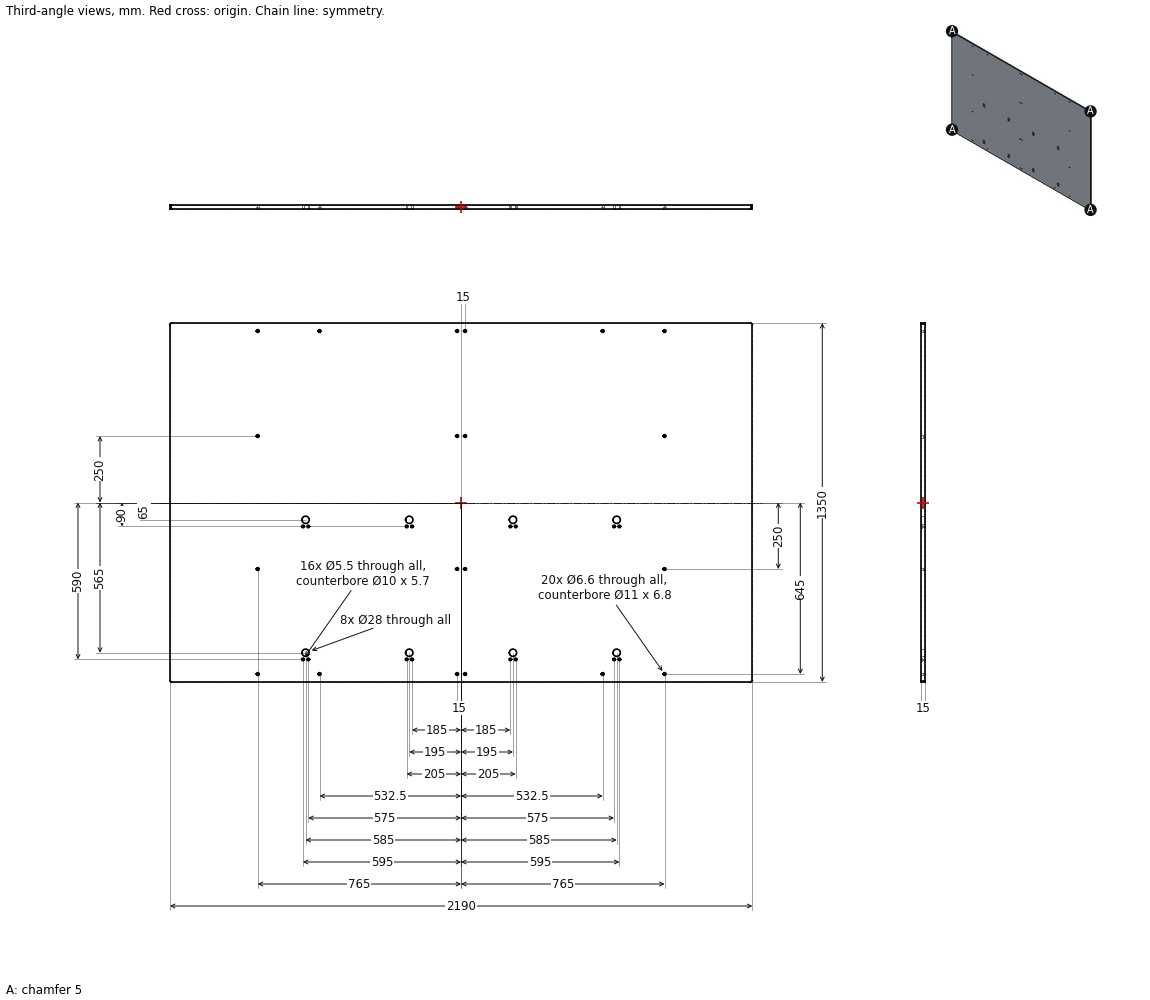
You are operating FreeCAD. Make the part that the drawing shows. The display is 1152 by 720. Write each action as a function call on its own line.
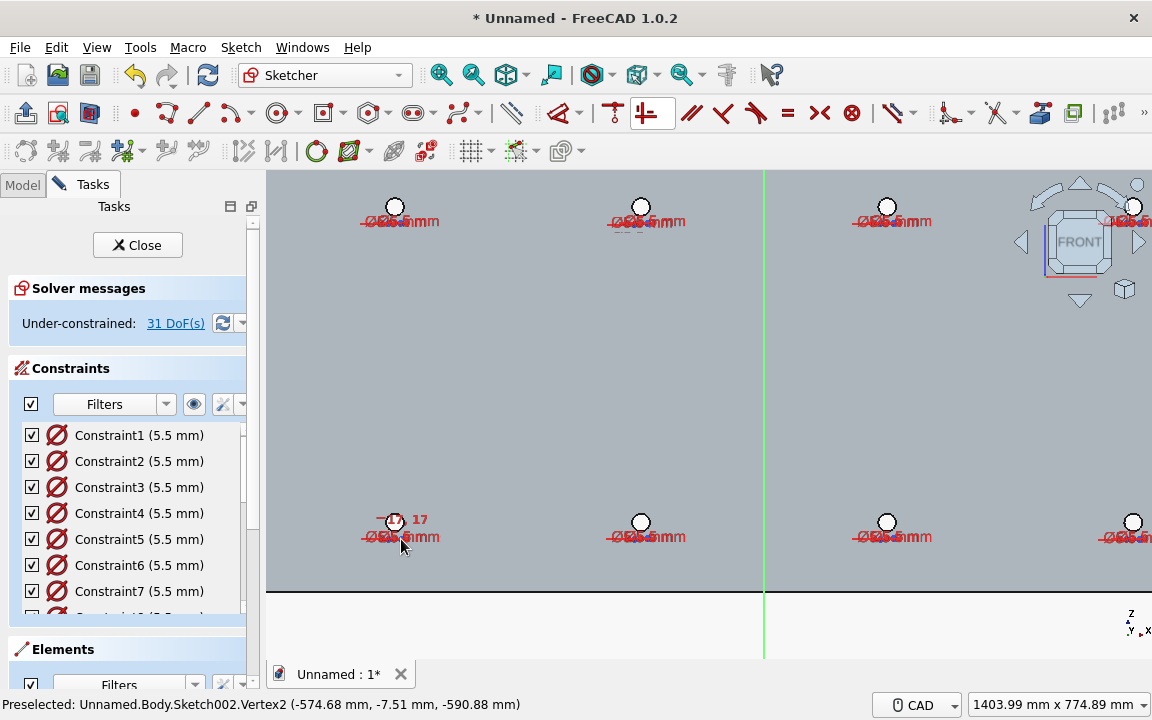
click(401, 539)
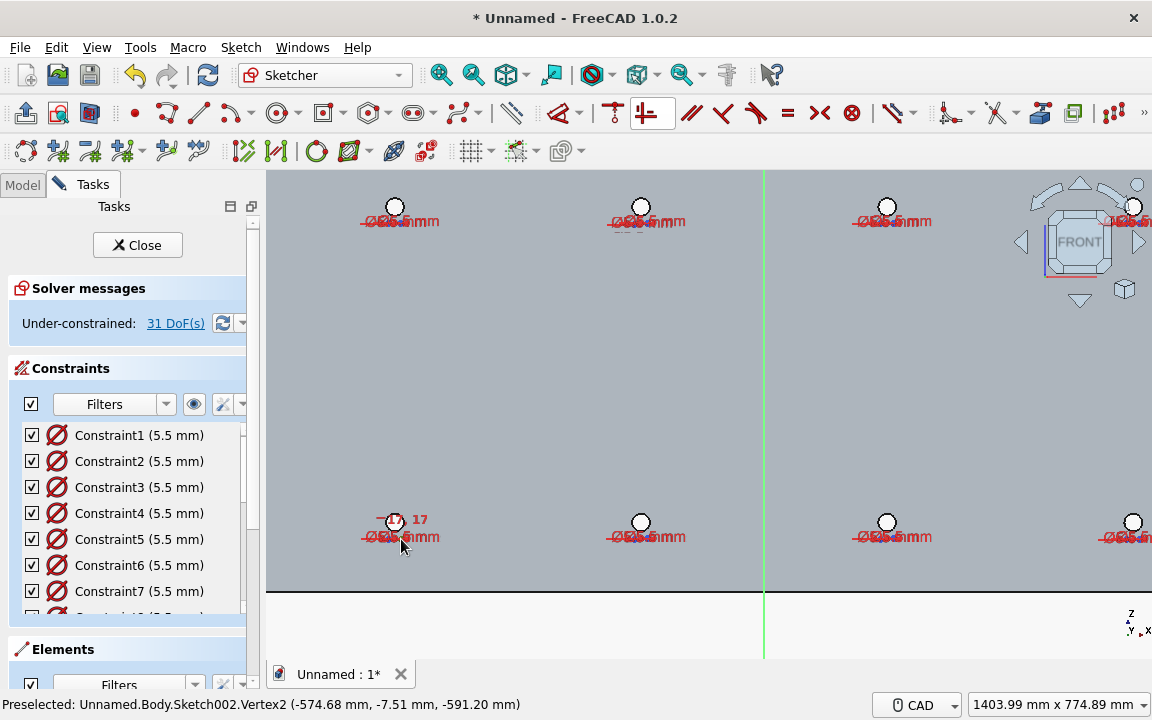
click(635, 539)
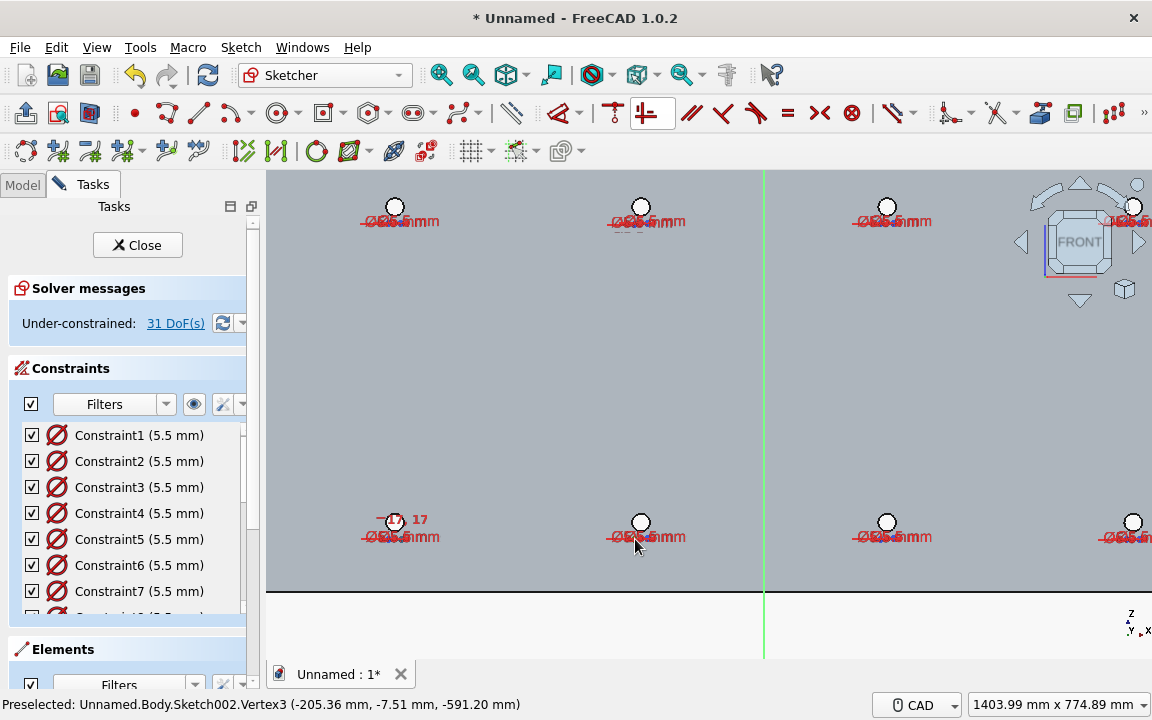
click(670, 114)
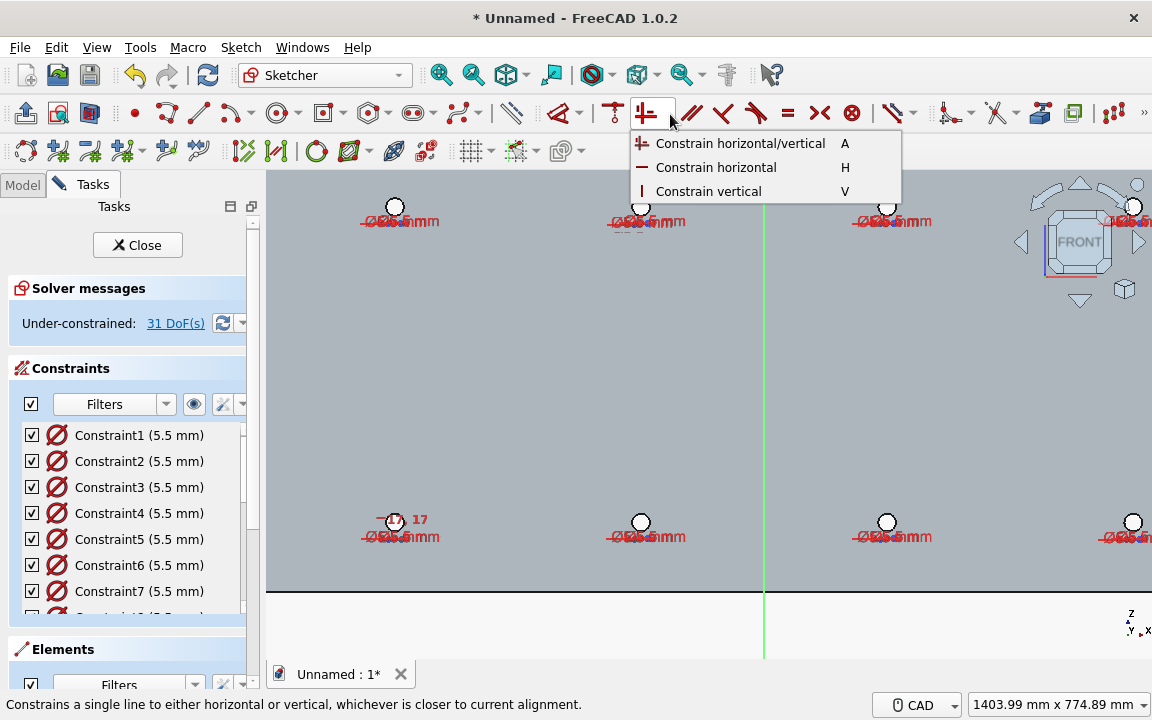
click(766, 167)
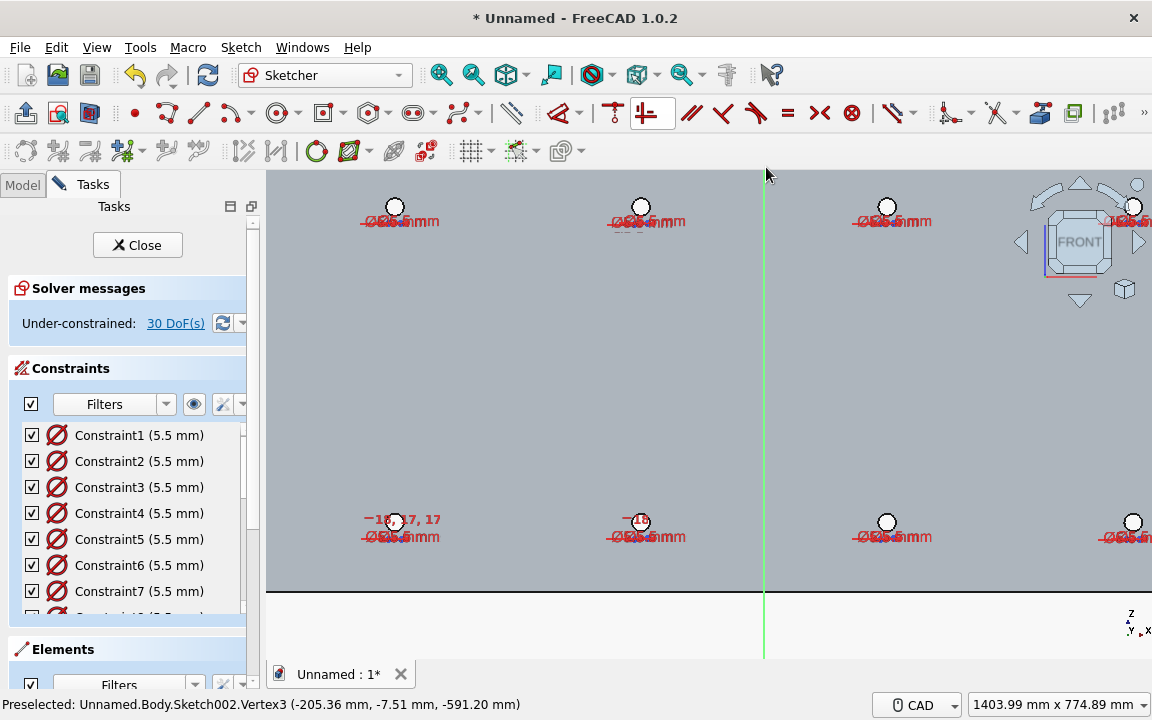
click(635, 539)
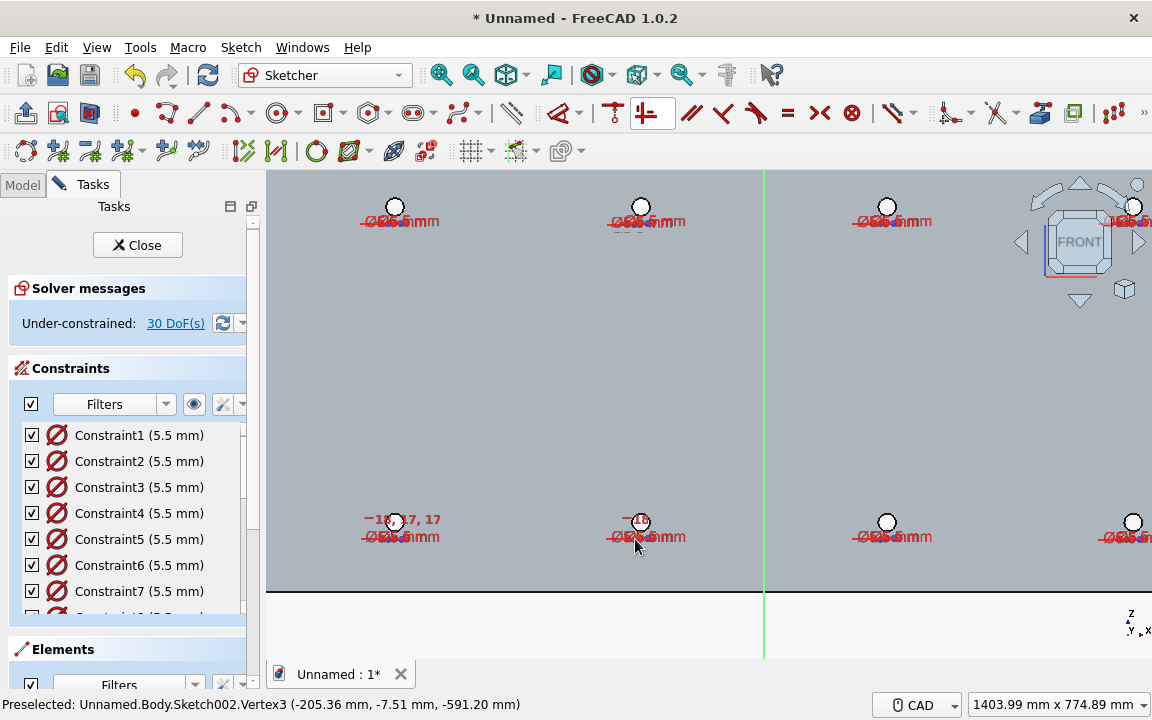
click(648, 539)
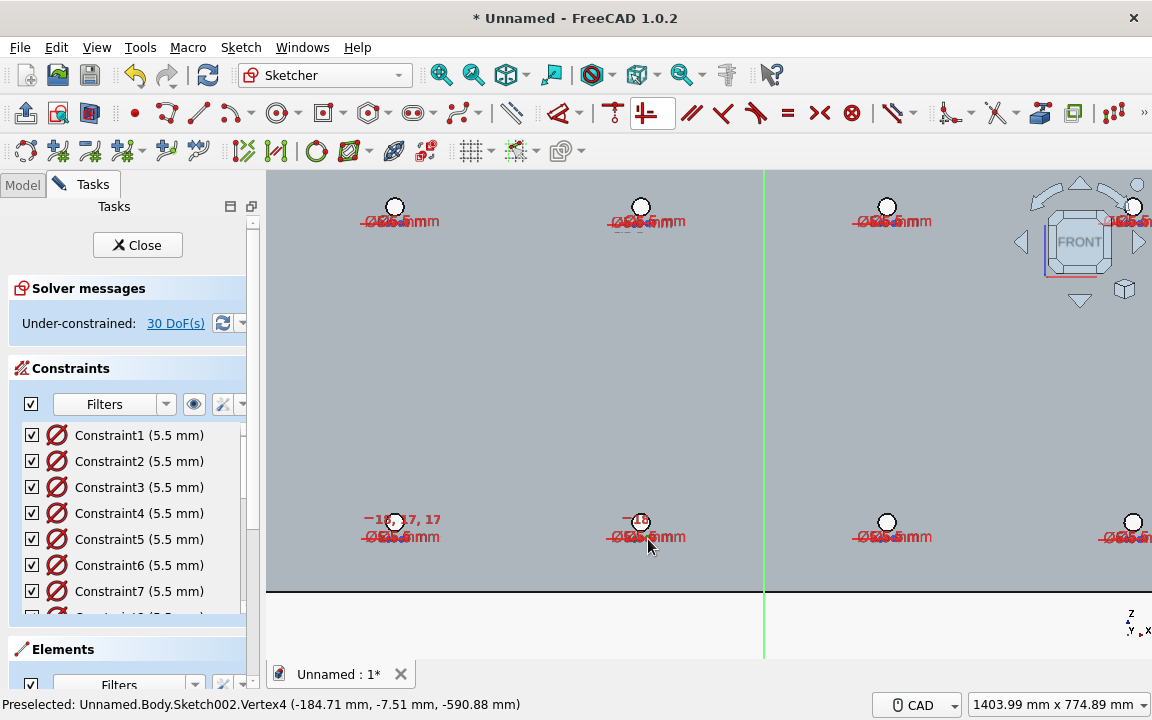
click(670, 114)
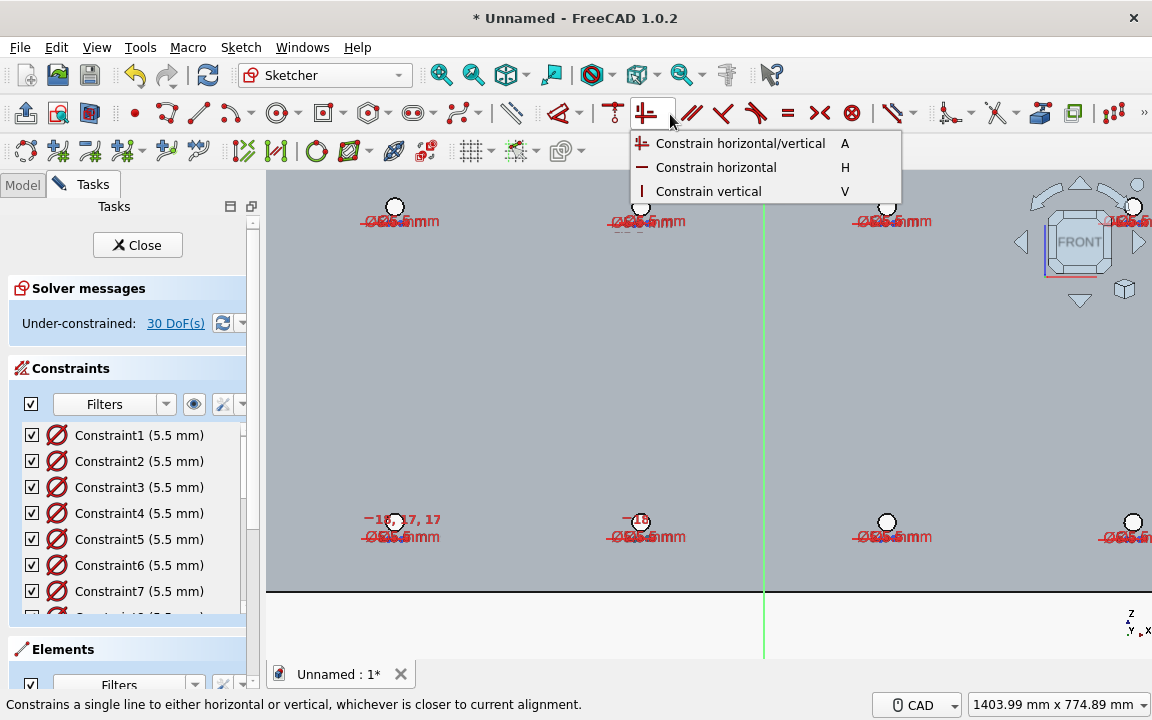
click(766, 167)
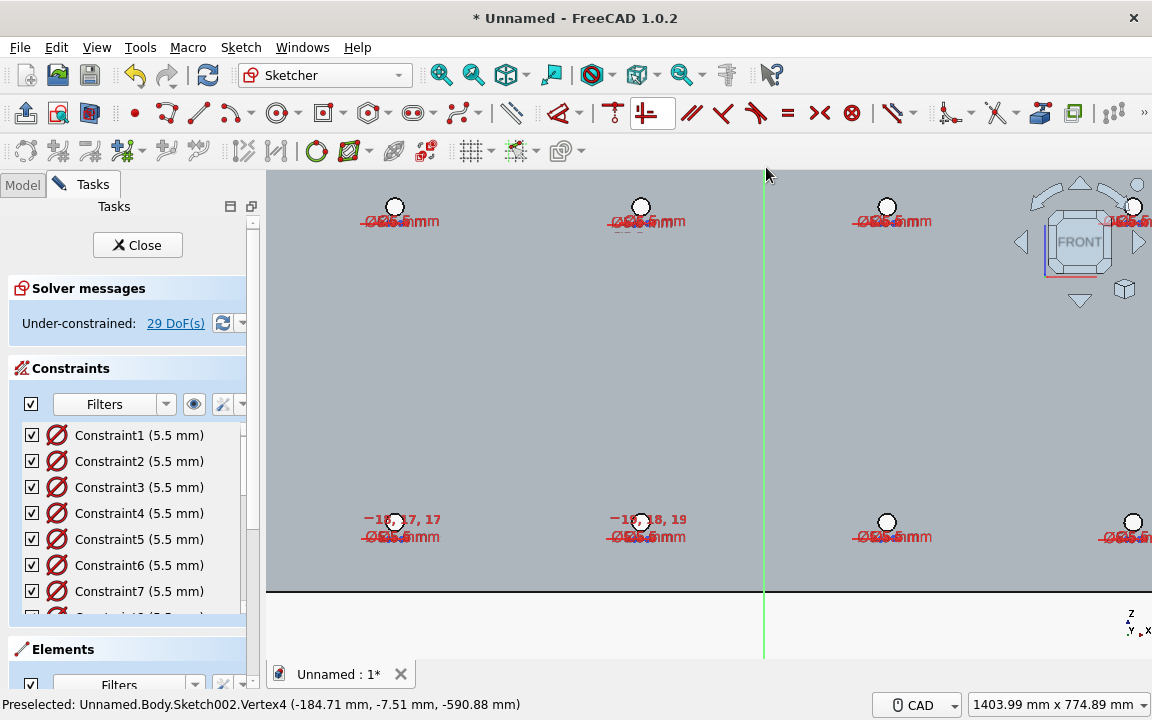
click(648, 539)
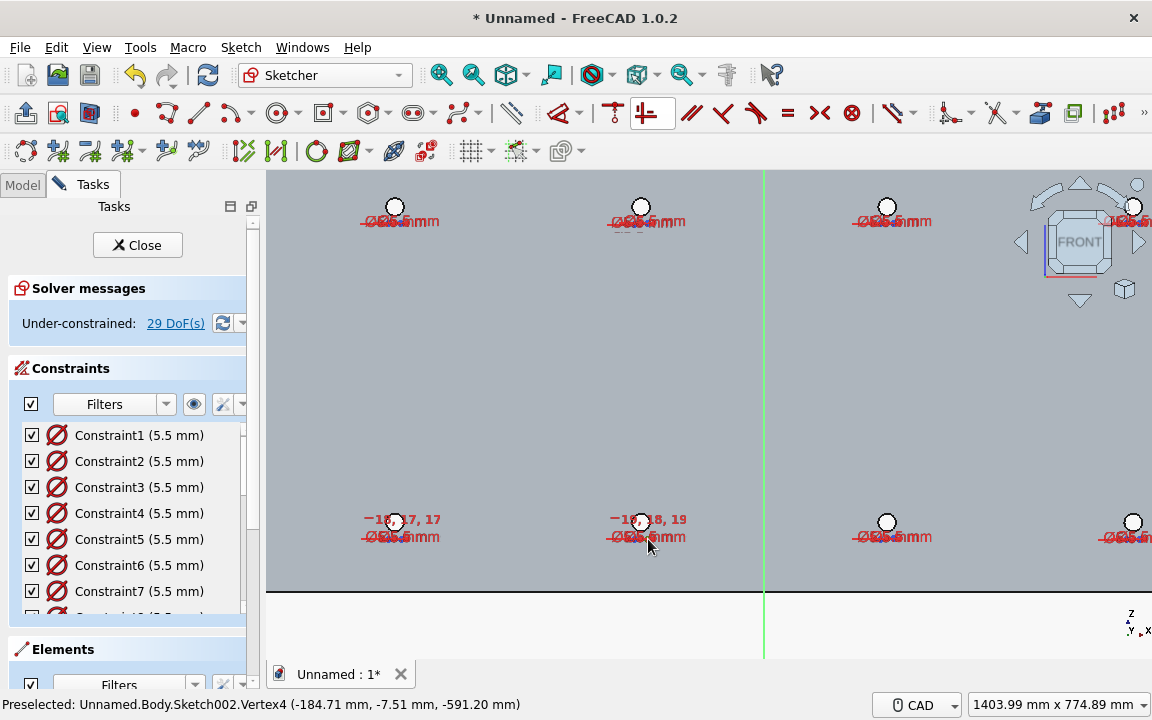
click(881, 539)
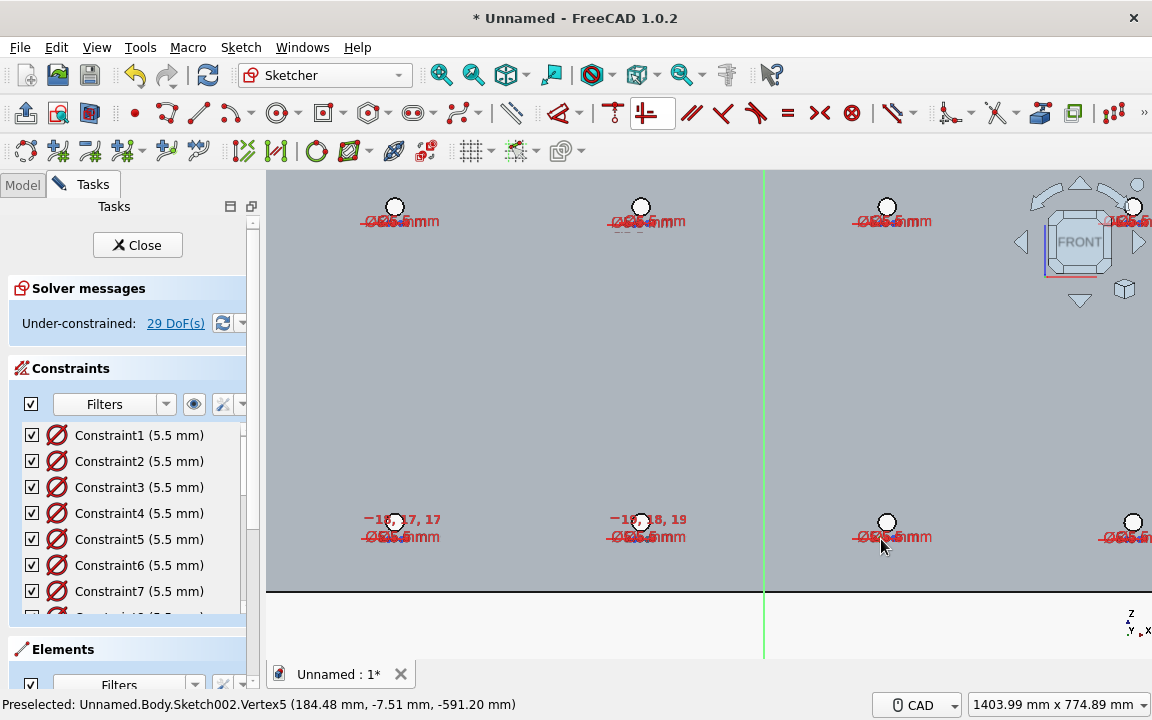
key(h)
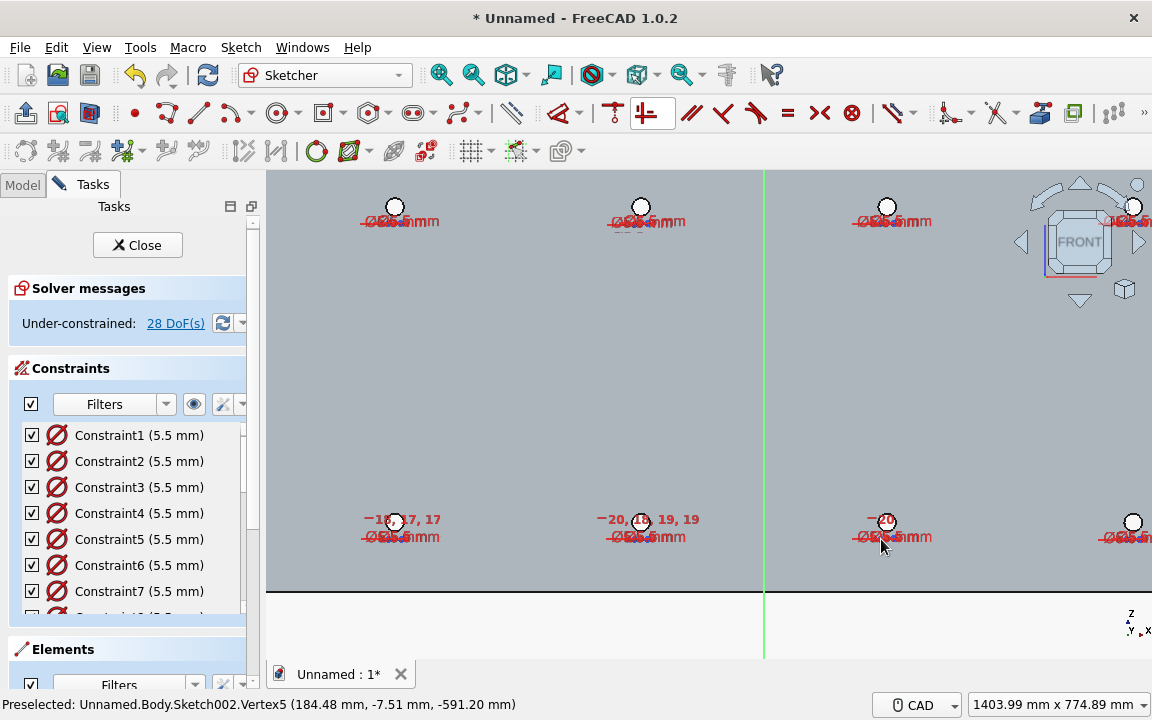
click(881, 539)